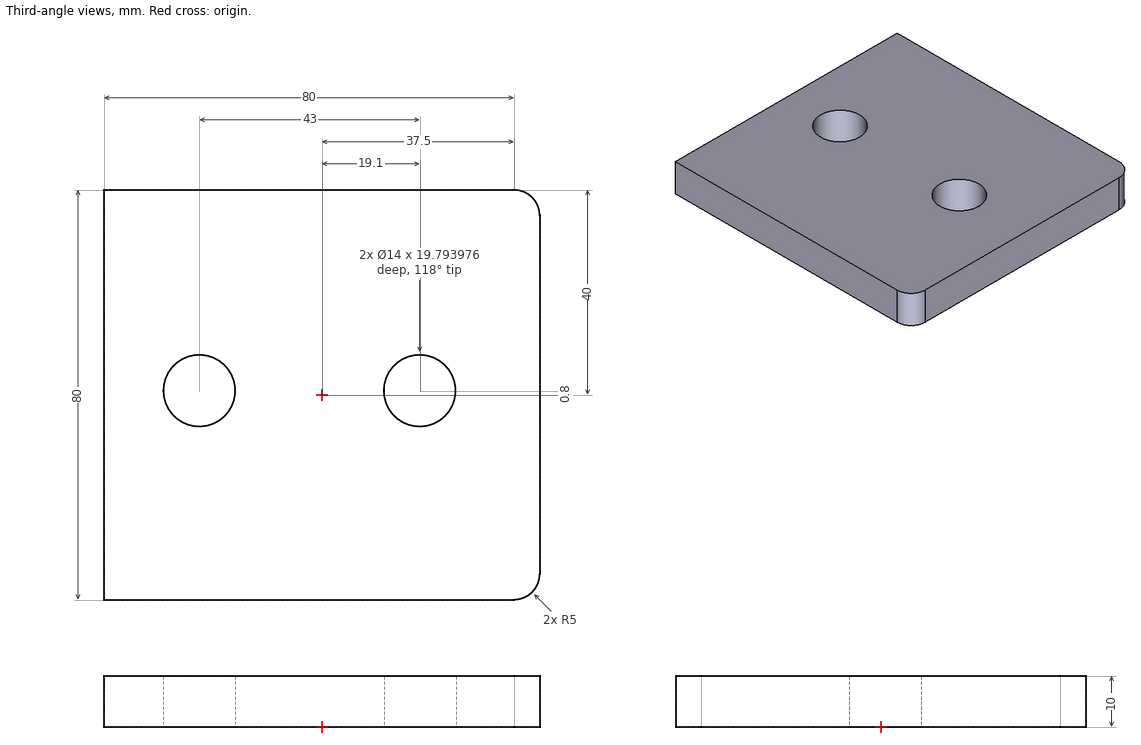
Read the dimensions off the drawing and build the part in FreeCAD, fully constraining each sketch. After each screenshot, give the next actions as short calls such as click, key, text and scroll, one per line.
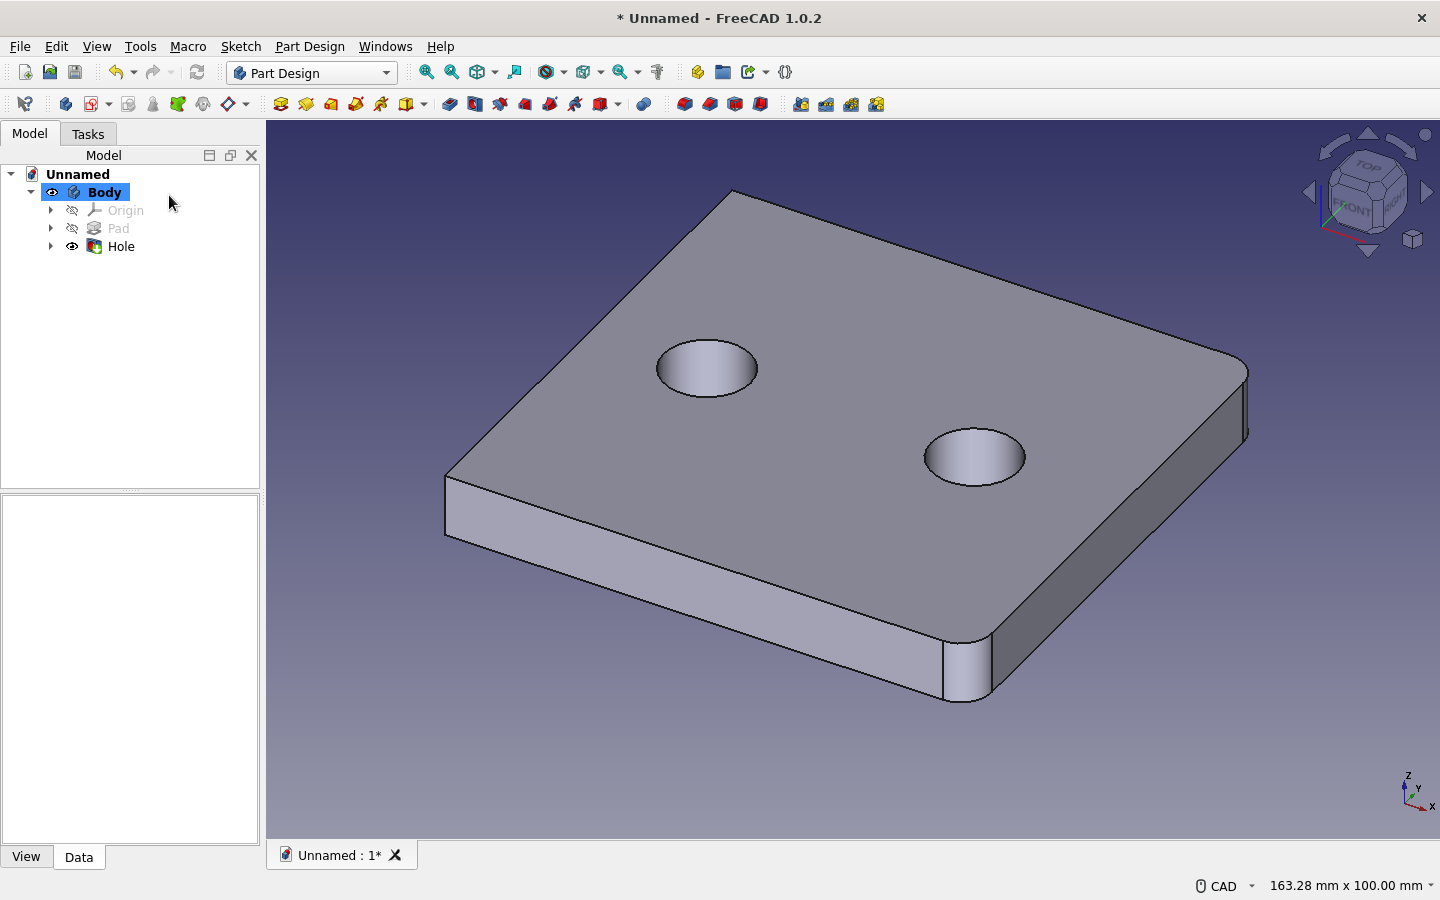
key(0)